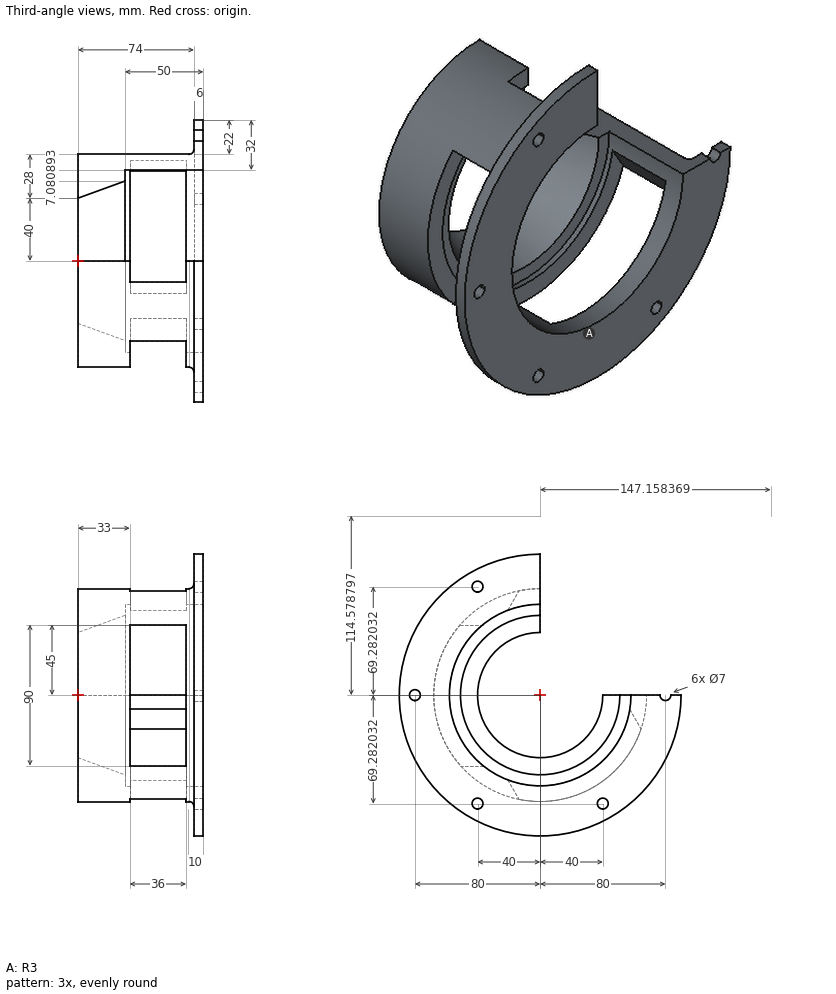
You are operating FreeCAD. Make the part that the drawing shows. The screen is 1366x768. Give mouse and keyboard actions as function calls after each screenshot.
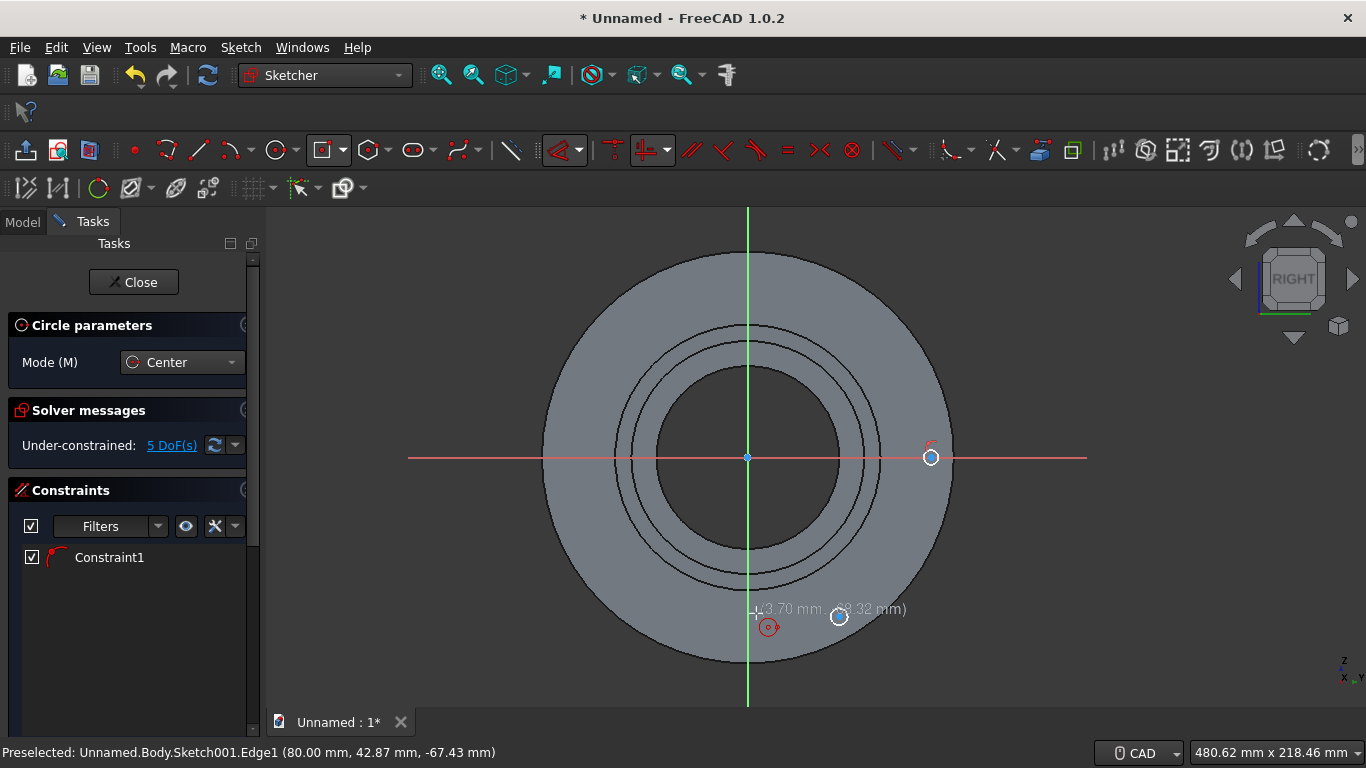
click(656, 616)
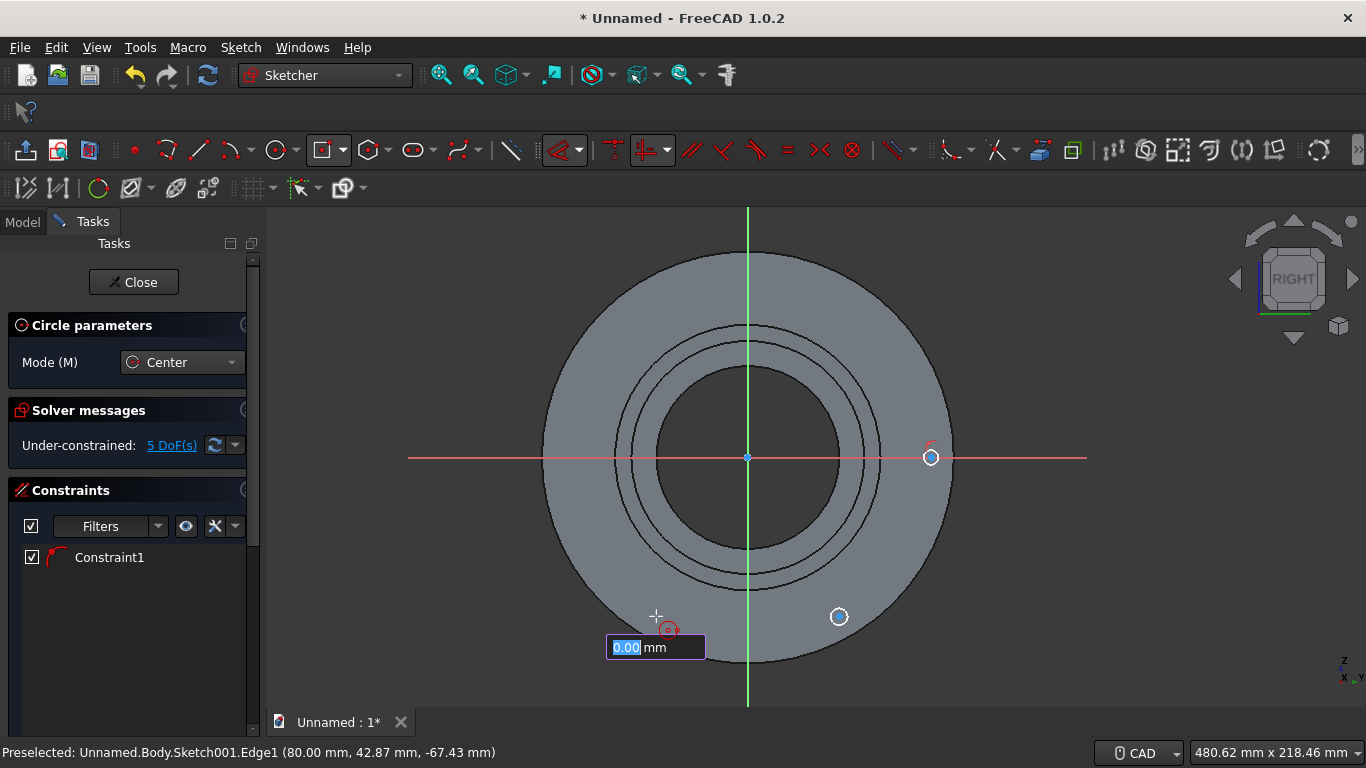
scroll(662, 610, up, 4)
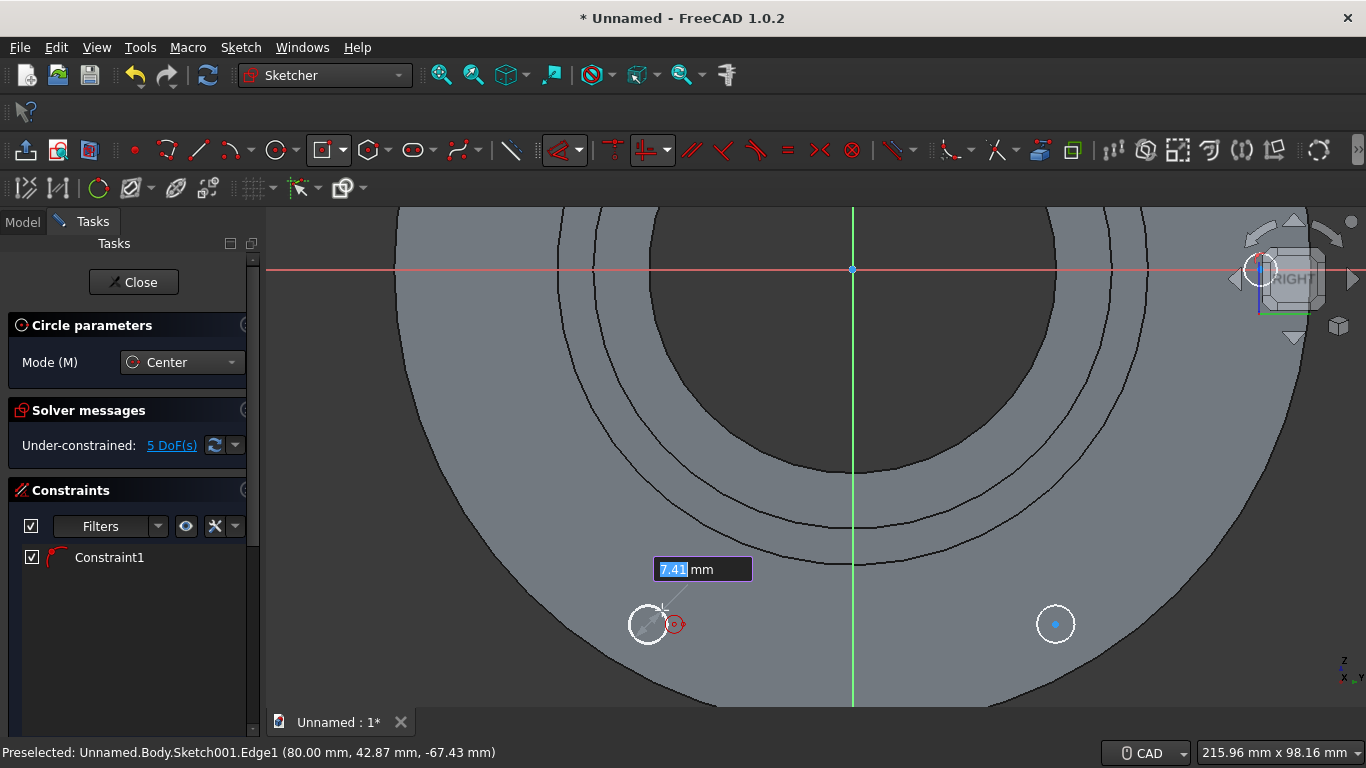
click(661, 610)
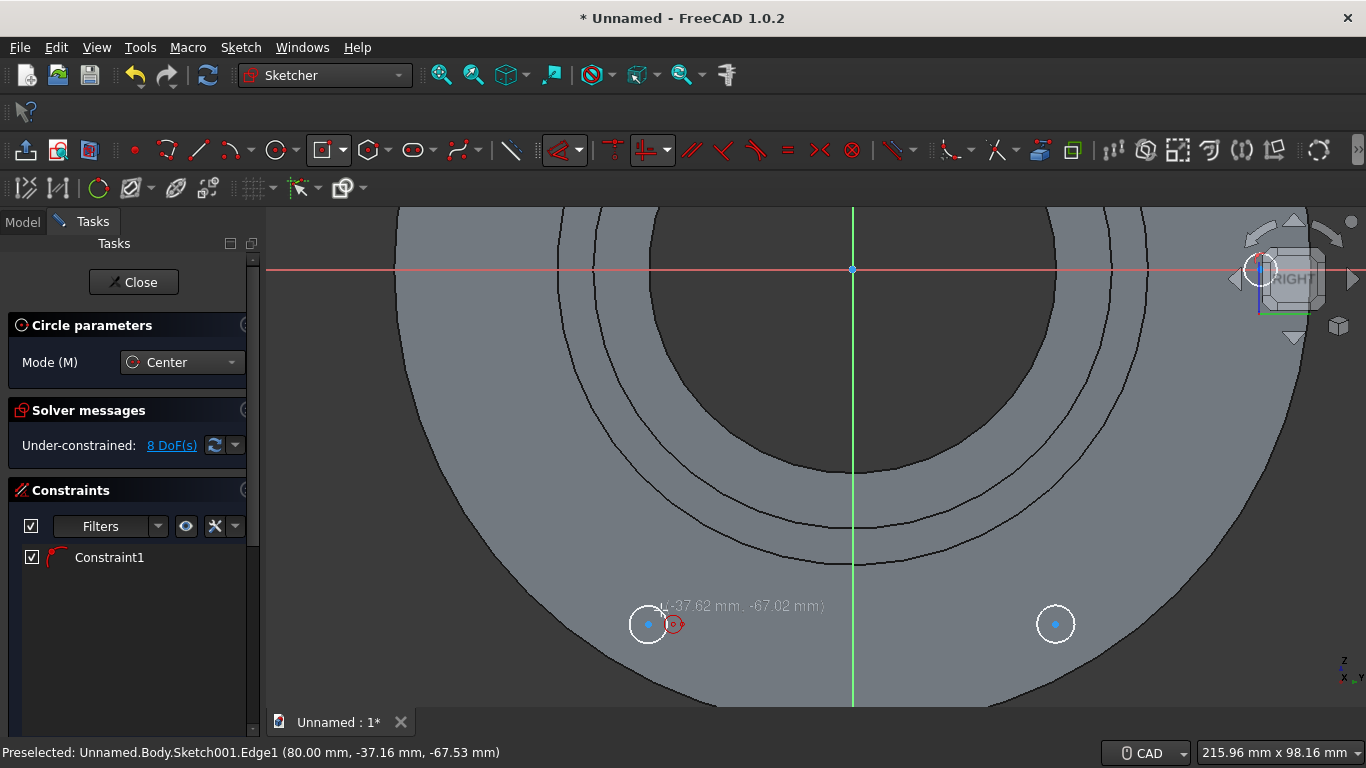
scroll(445, 270, up, 2)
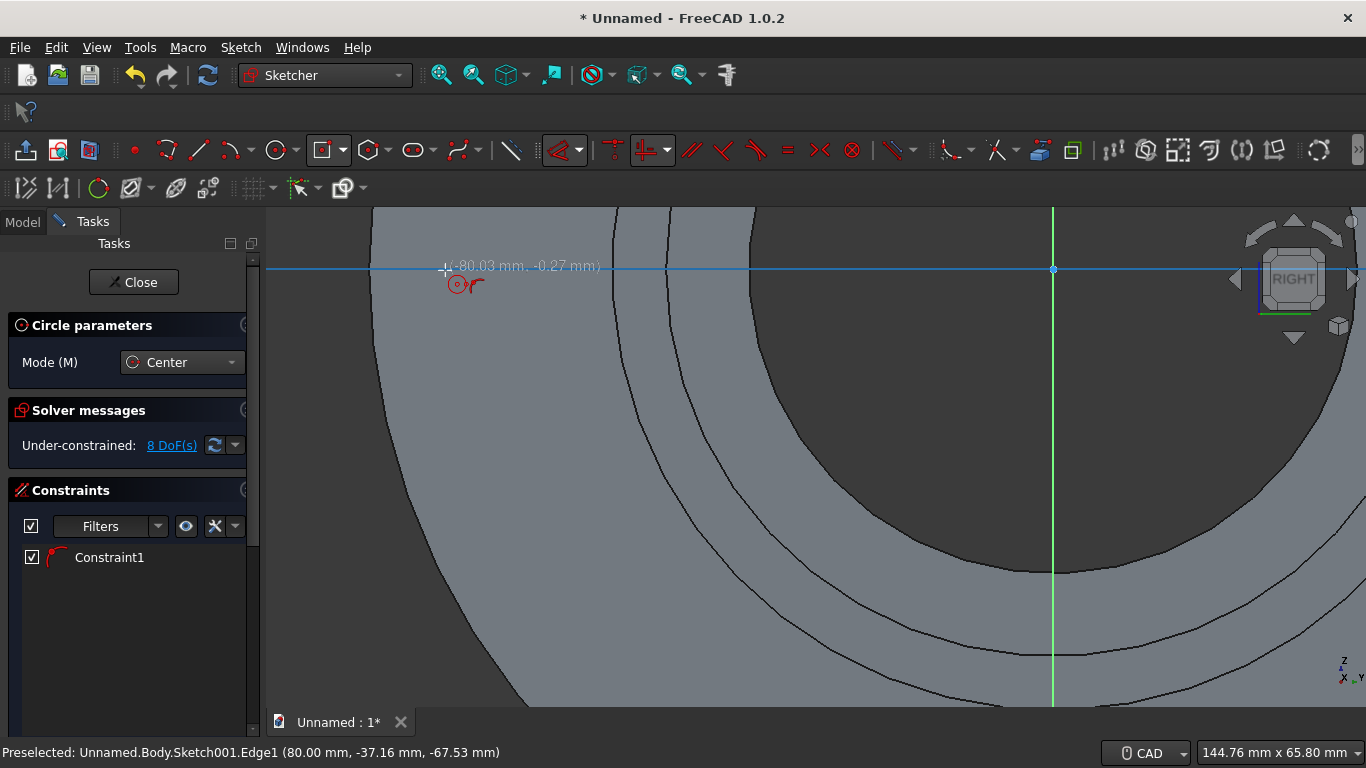
scroll(616, 538, down, 6)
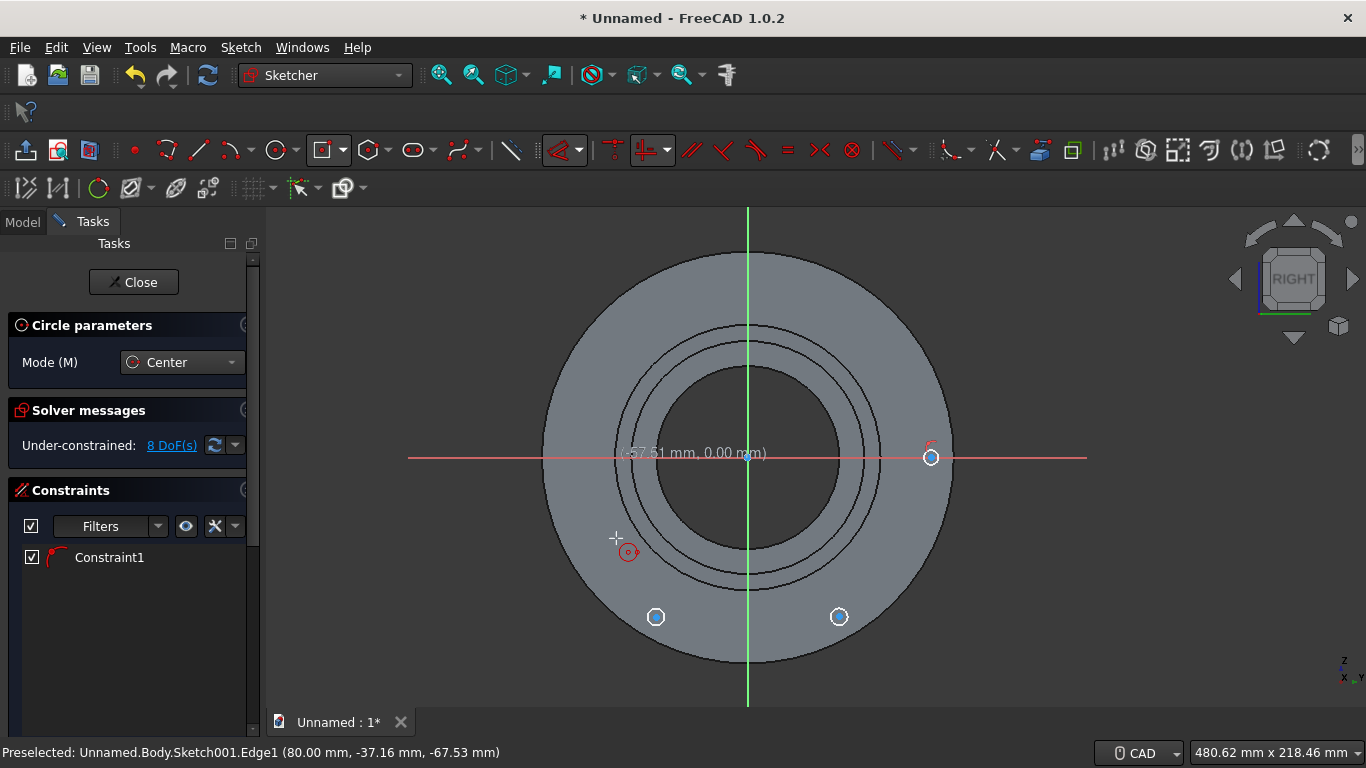
click(565, 458)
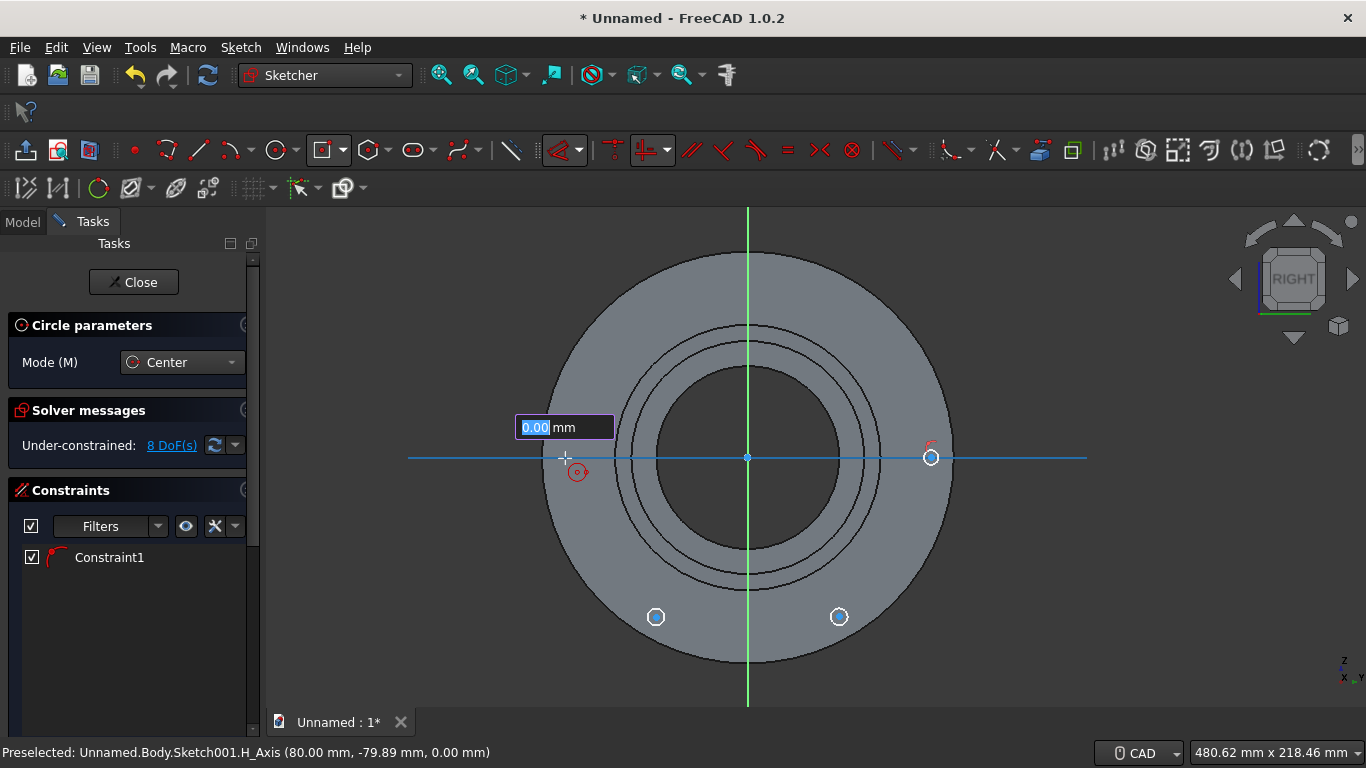
scroll(567, 450, up, 4)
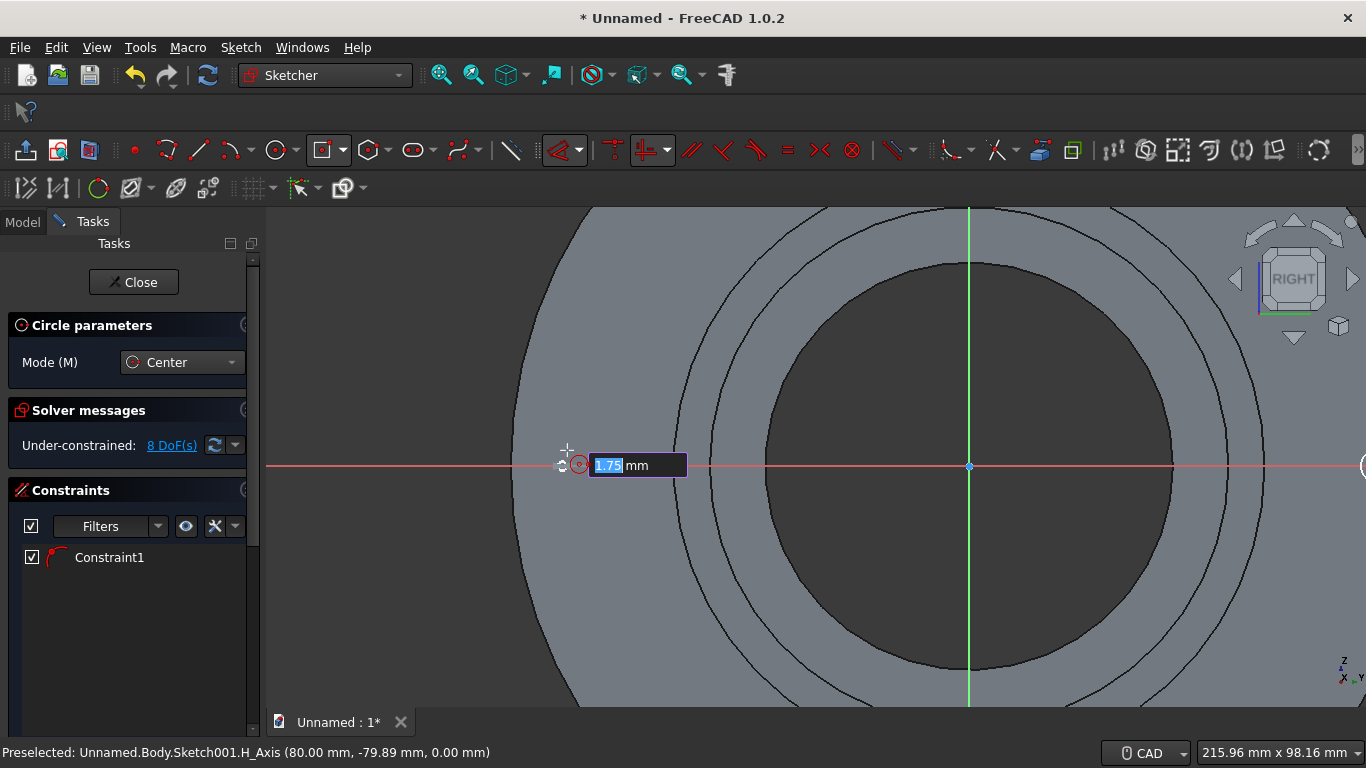
click(568, 449)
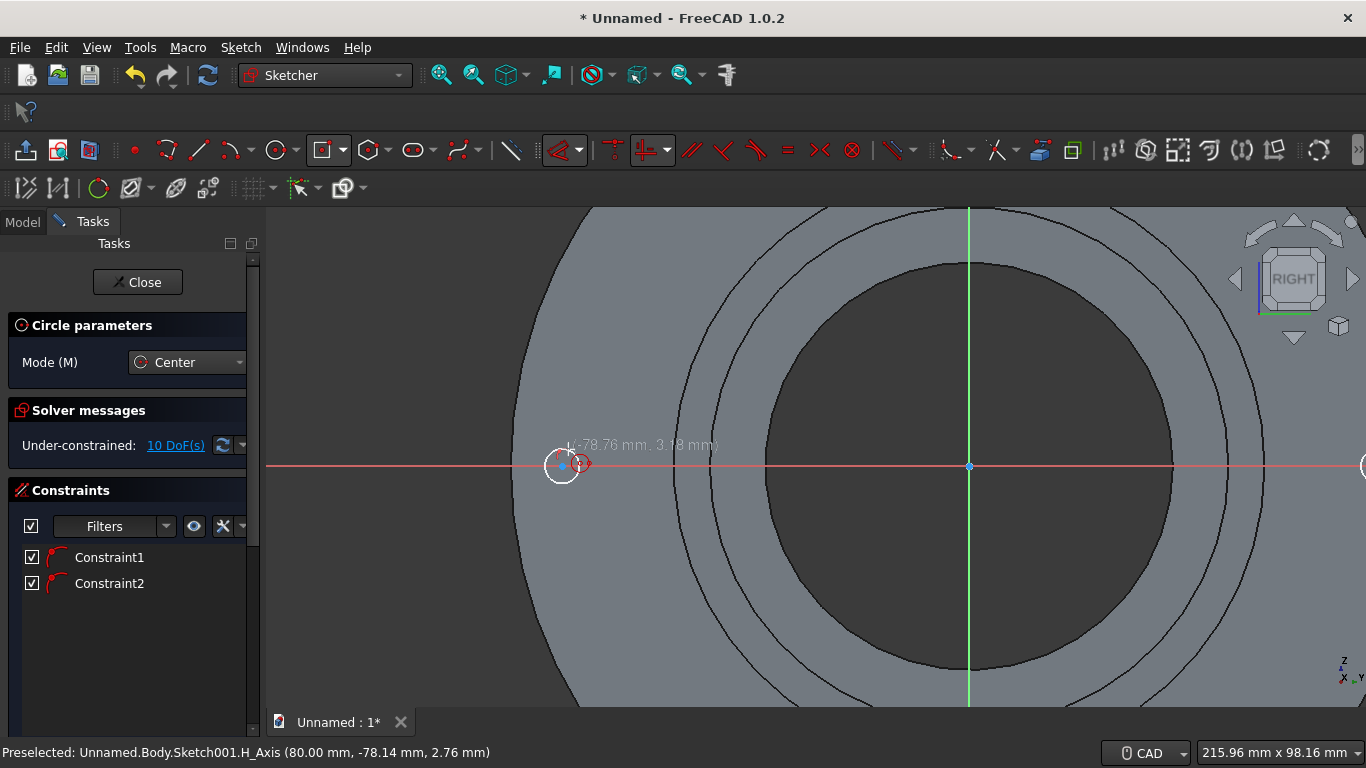
scroll(567, 449, down, 4)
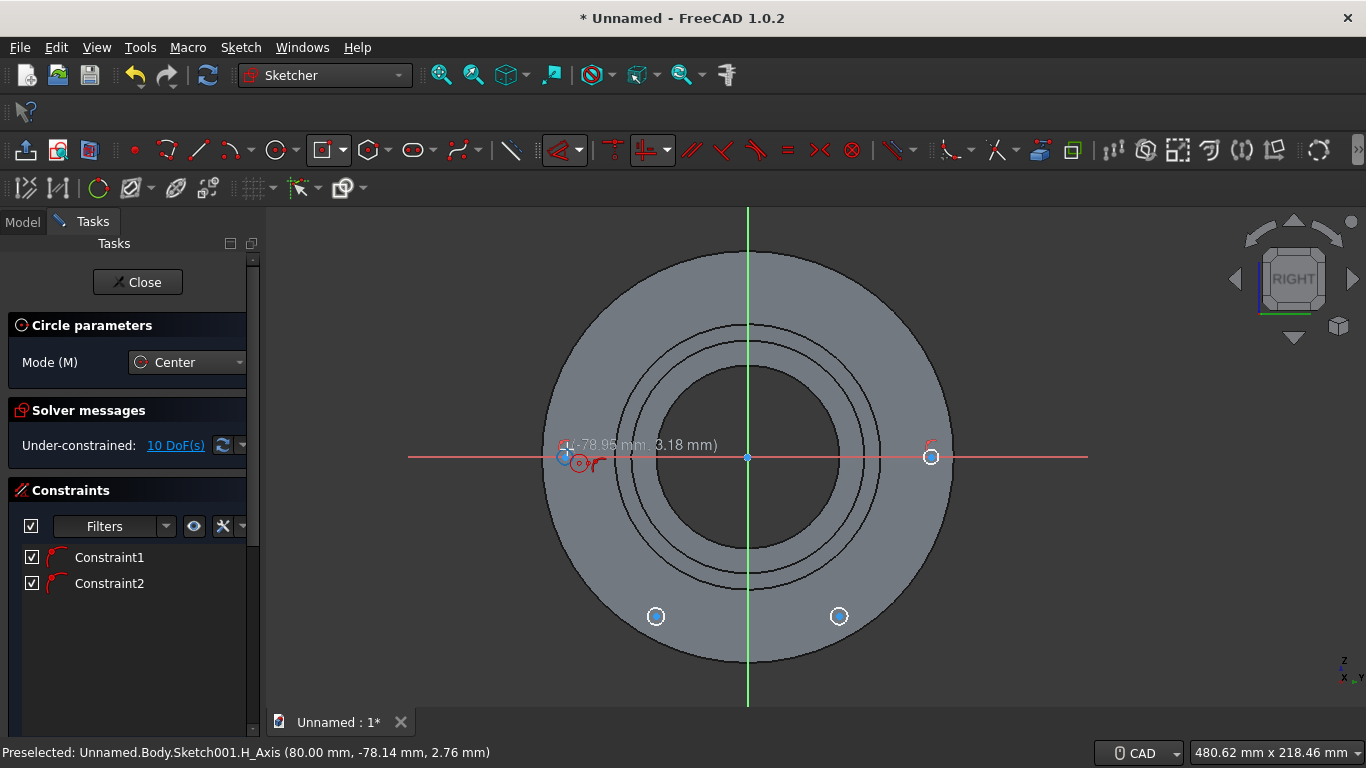
scroll(656, 298, up, 6)